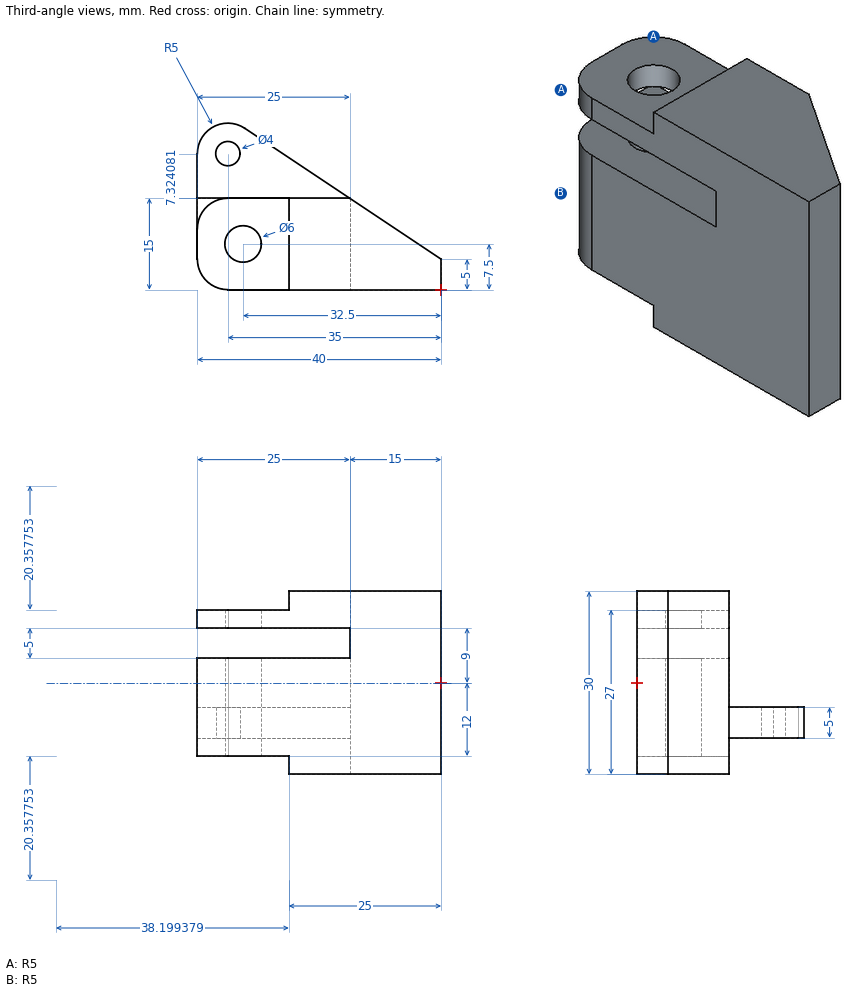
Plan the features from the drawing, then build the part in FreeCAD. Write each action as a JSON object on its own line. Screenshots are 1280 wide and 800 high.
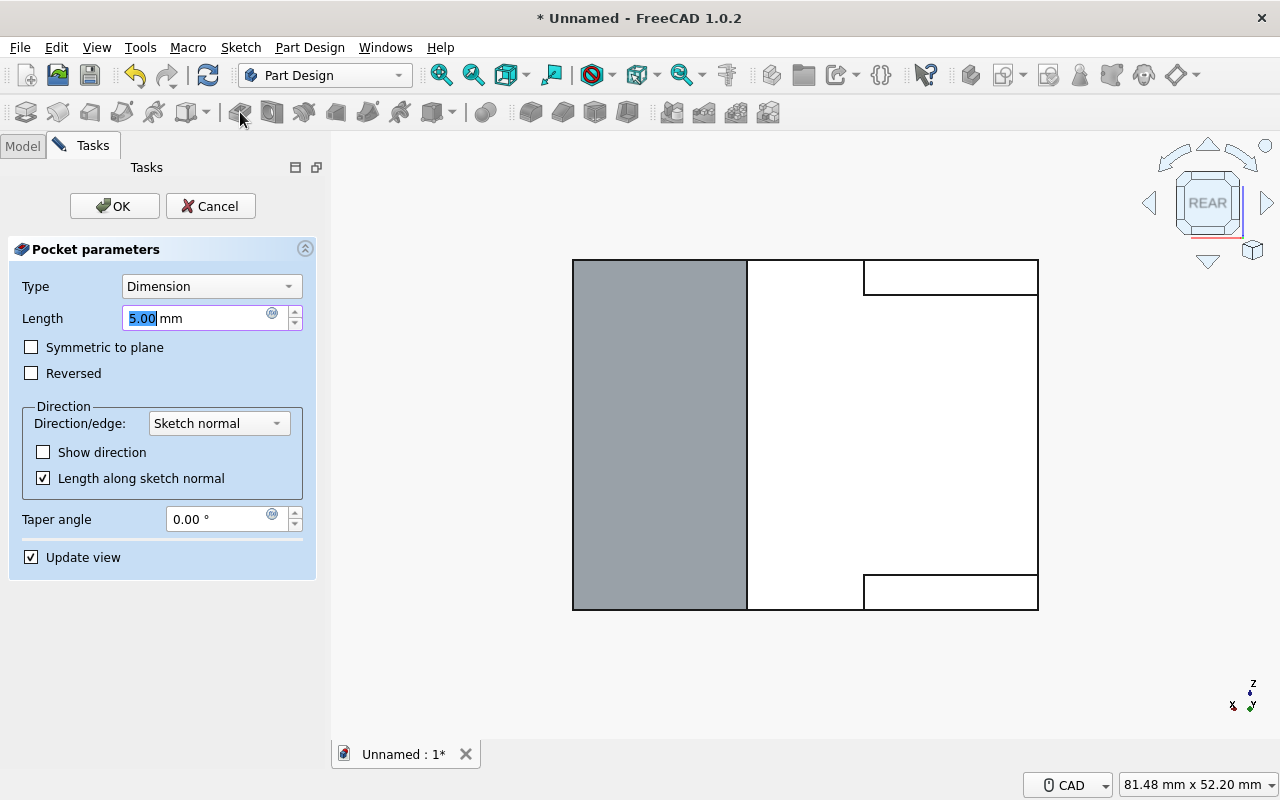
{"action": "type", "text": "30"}
{"action": "key", "text": "Tab"}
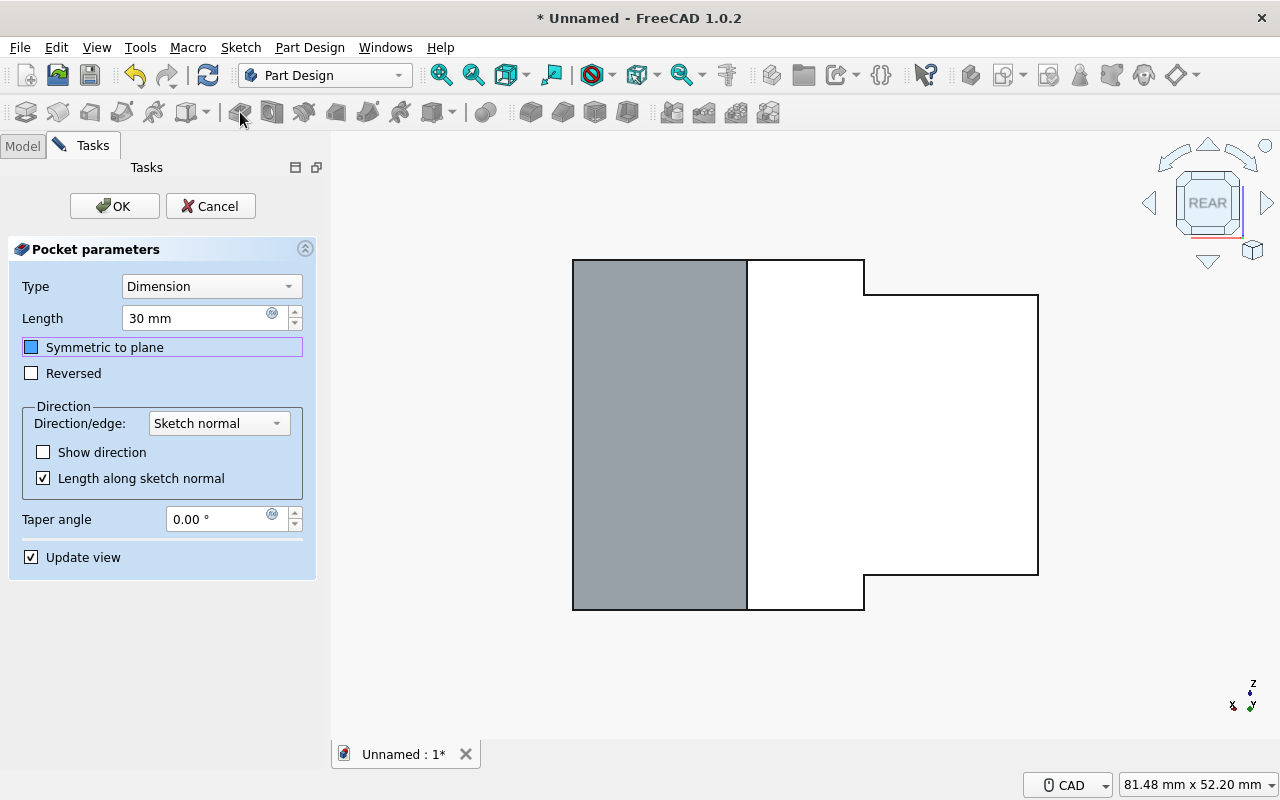
{"action": "left_click", "coordinate": [115, 206]}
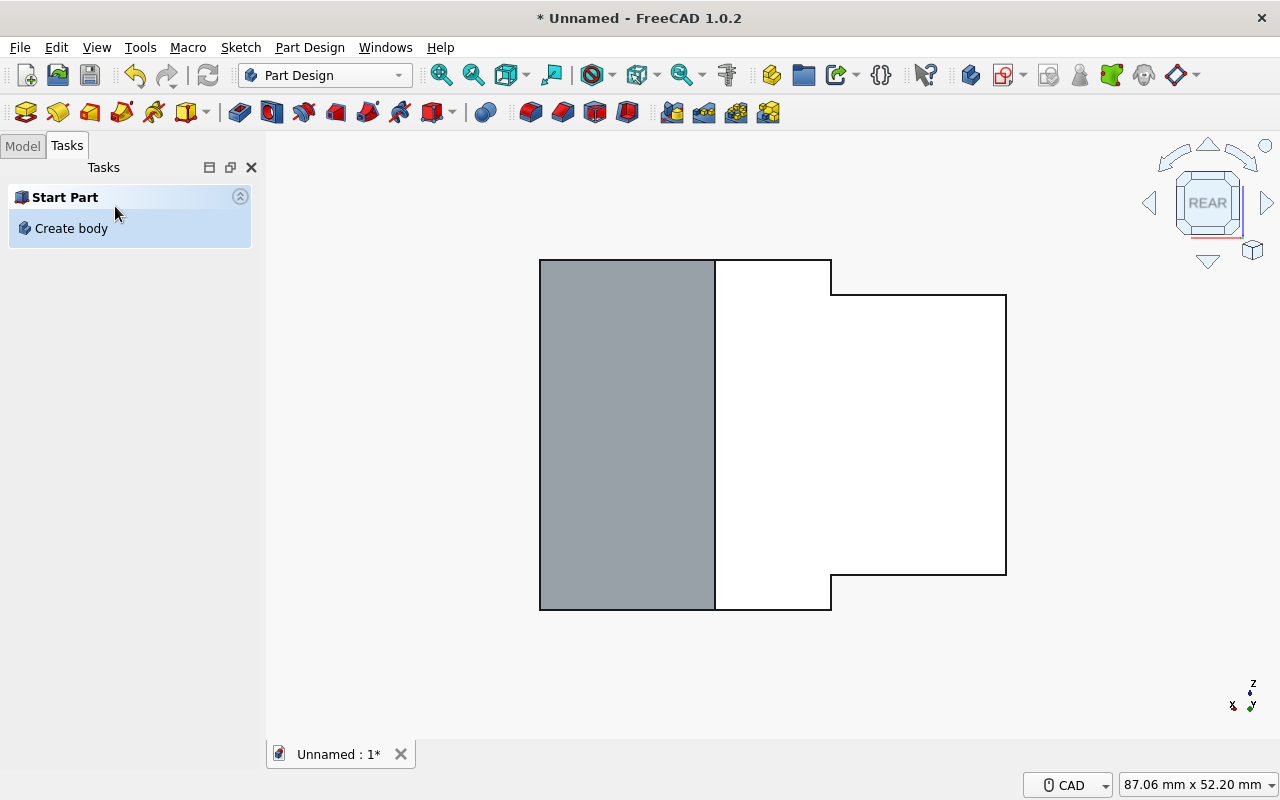
{"action": "left_click", "coordinate": [860, 434]}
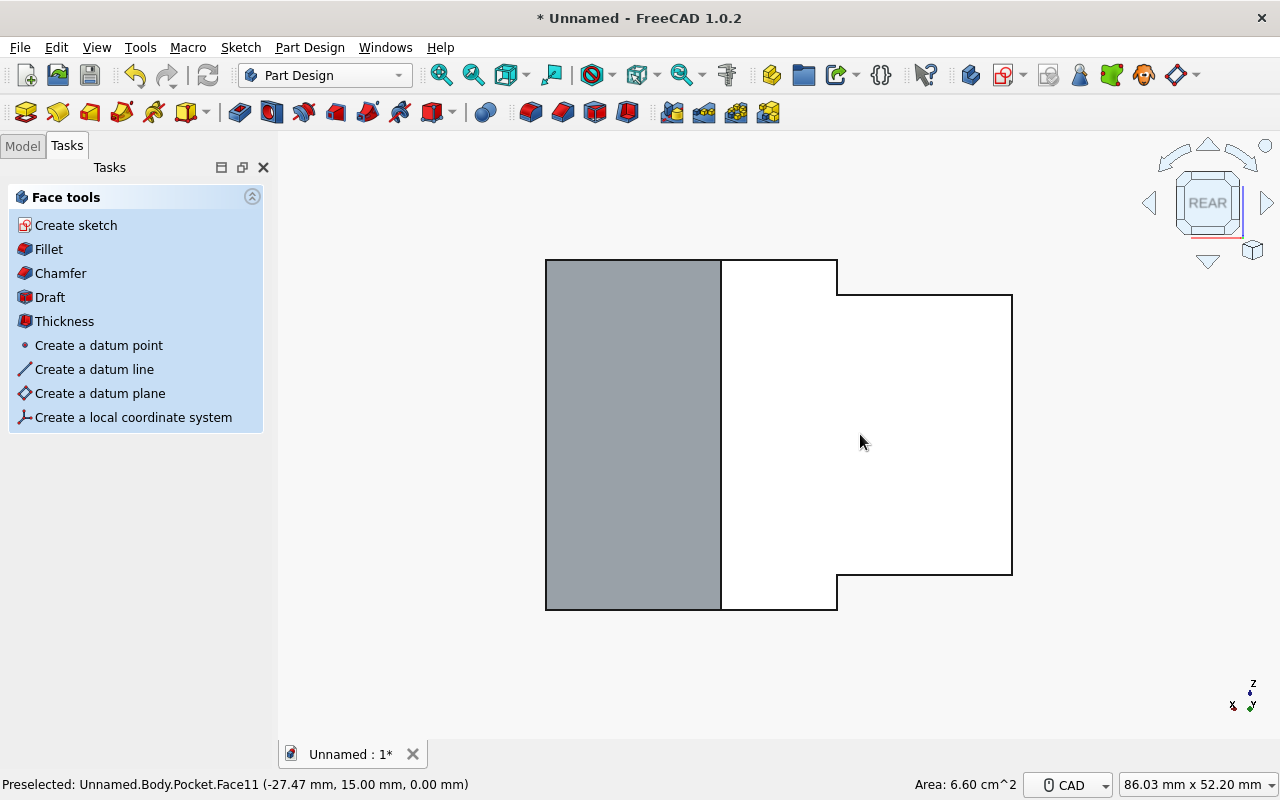
{"action": "left_click", "coordinate": [1004, 76]}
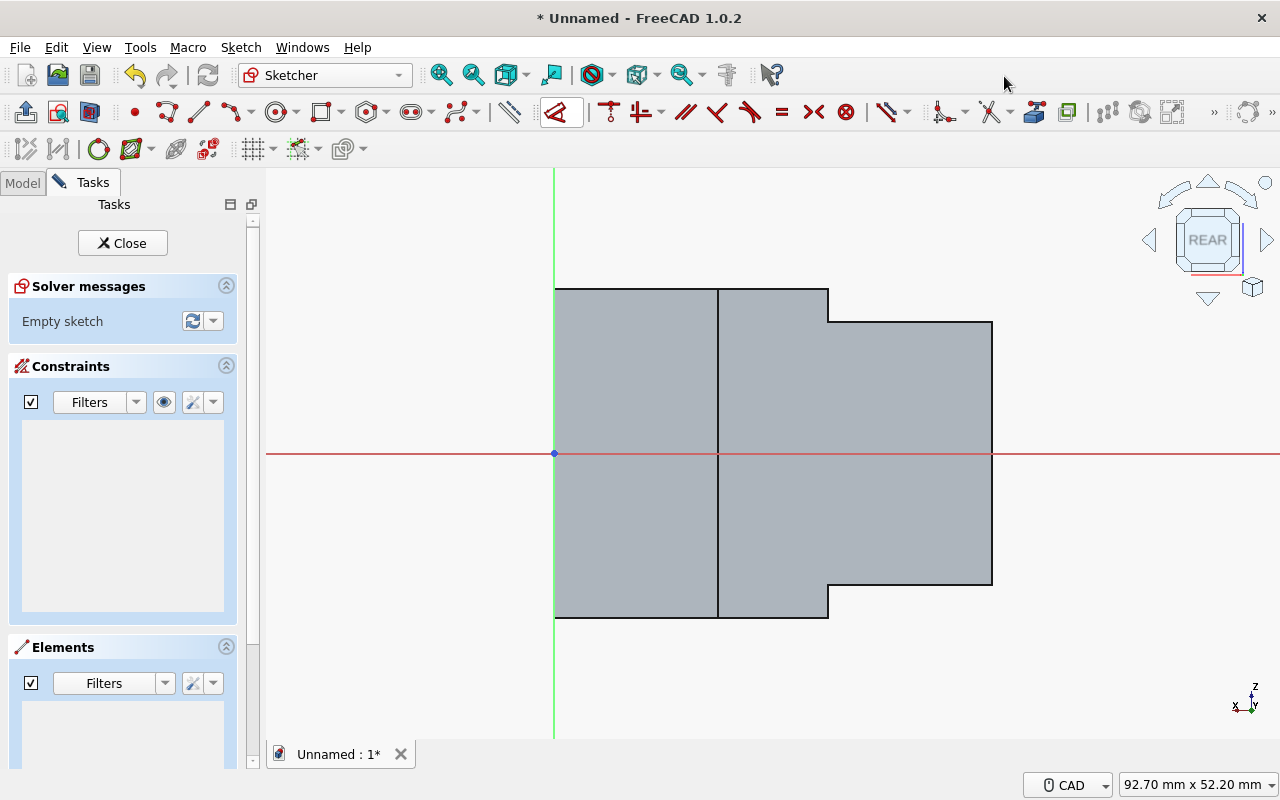
{"action": "left_click", "coordinate": [322, 112]}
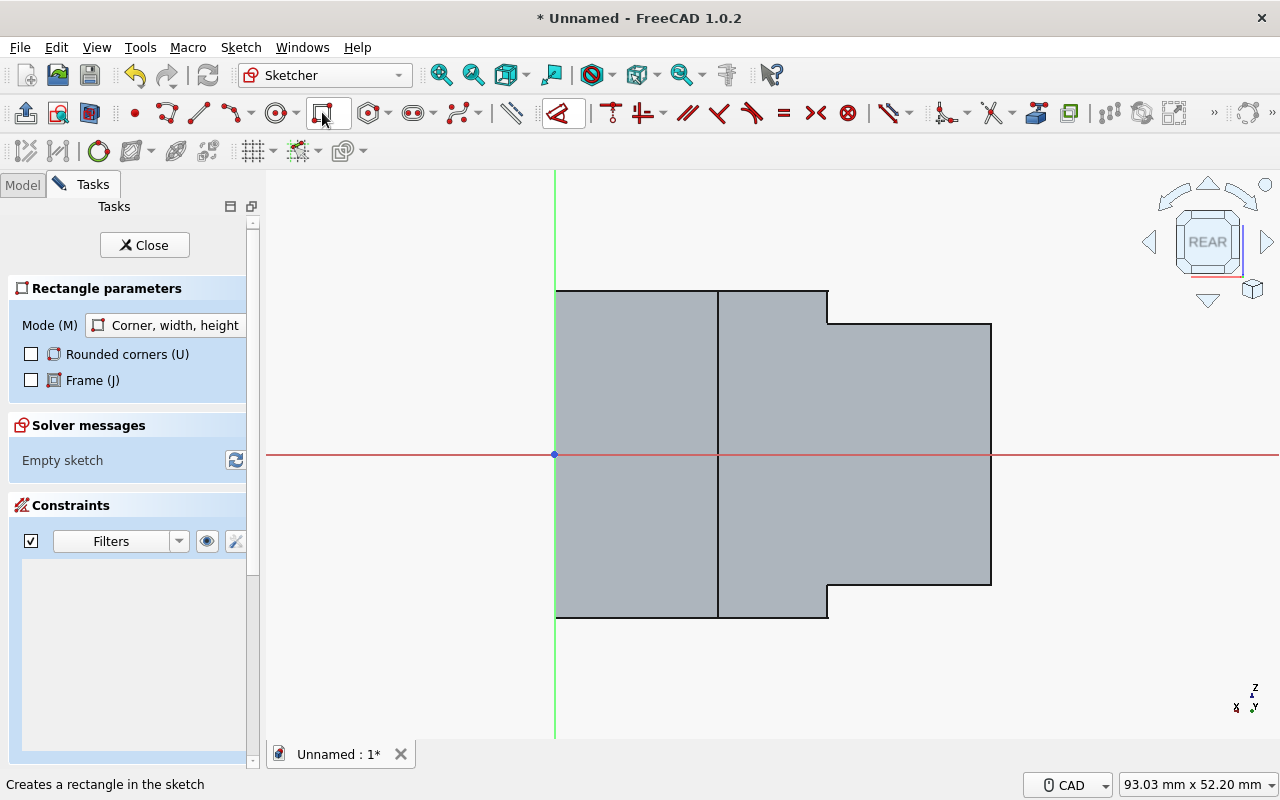
{"action": "left_click", "coordinate": [718, 356]}
{"action": "mouse_move", "coordinate": [991, 411]}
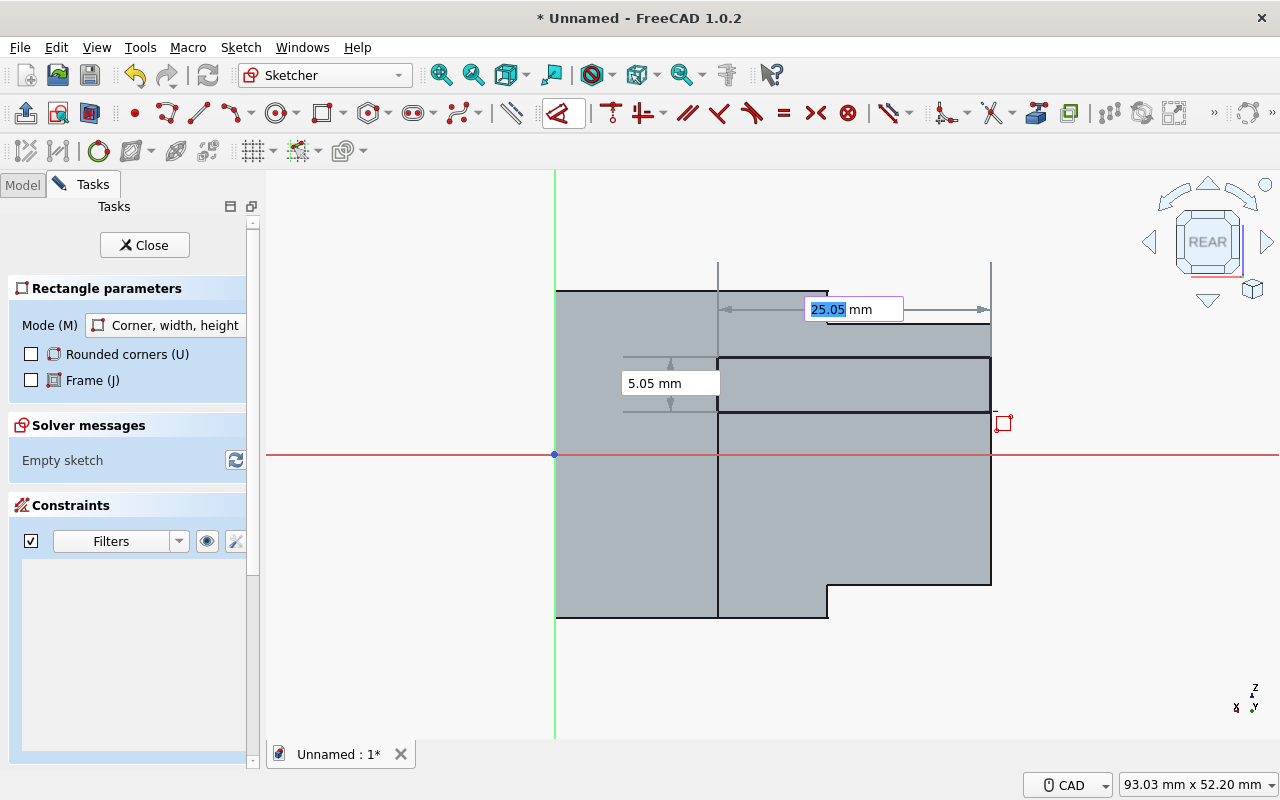
{"action": "type", "text": "25"}
{"action": "key", "text": "Tab"}
{"action": "type", "text": "5"}
{"action": "key", "text": "Return"}
{"action": "key", "text": "Escape"}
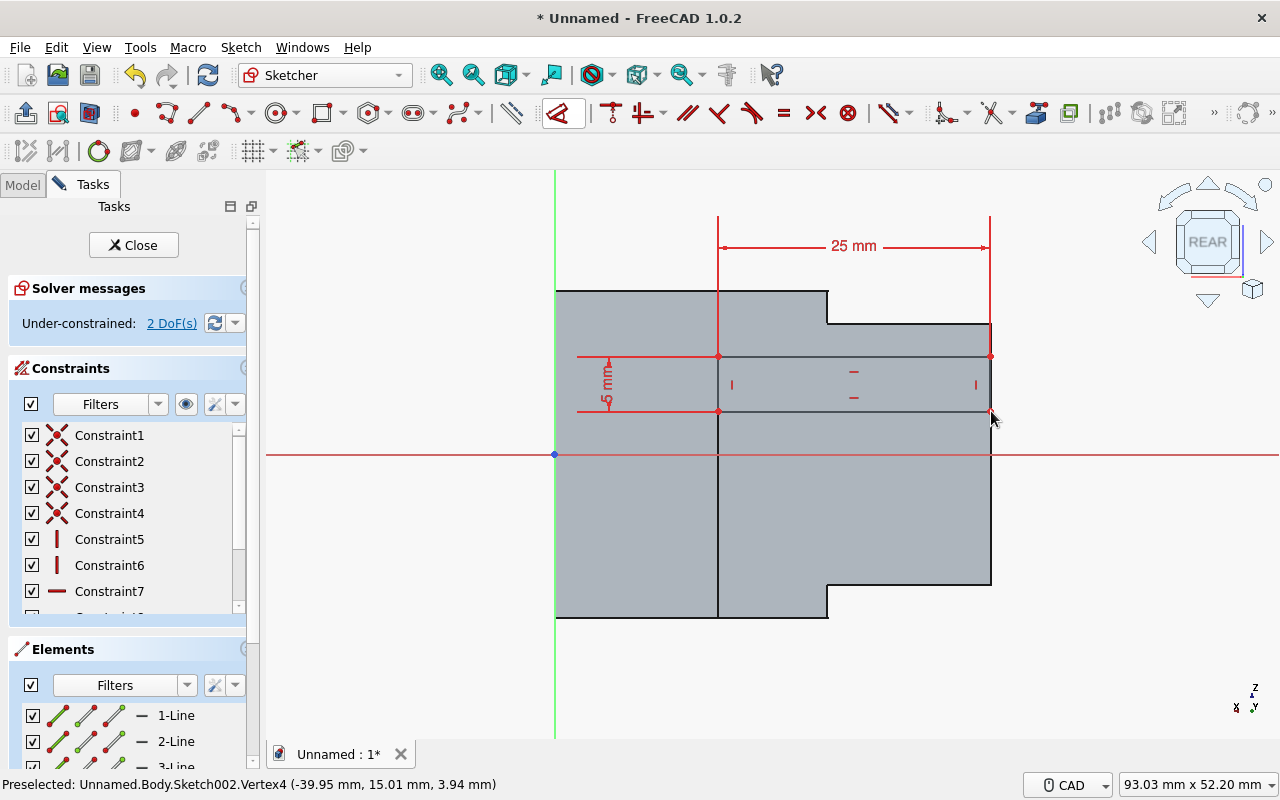
{"action": "left_click", "coordinate": [718, 357]}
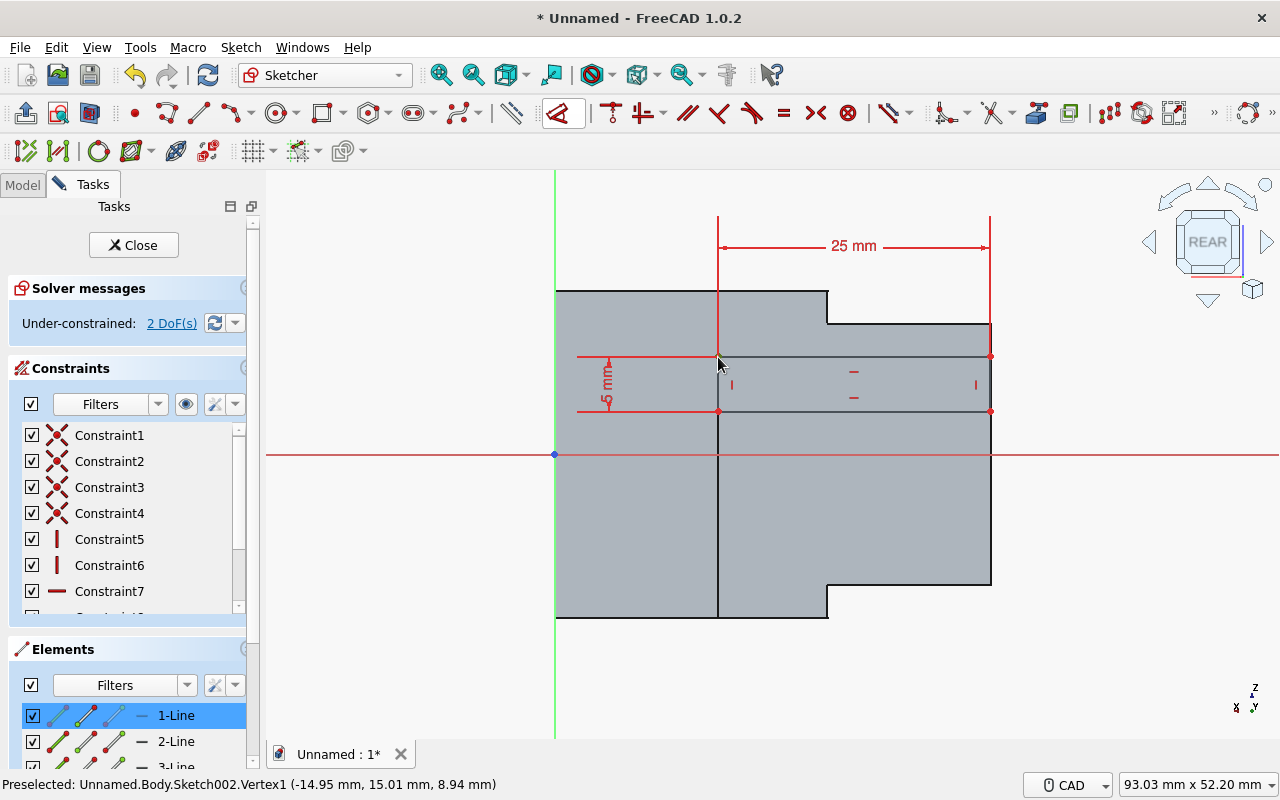
{"action": "key", "text": "i"}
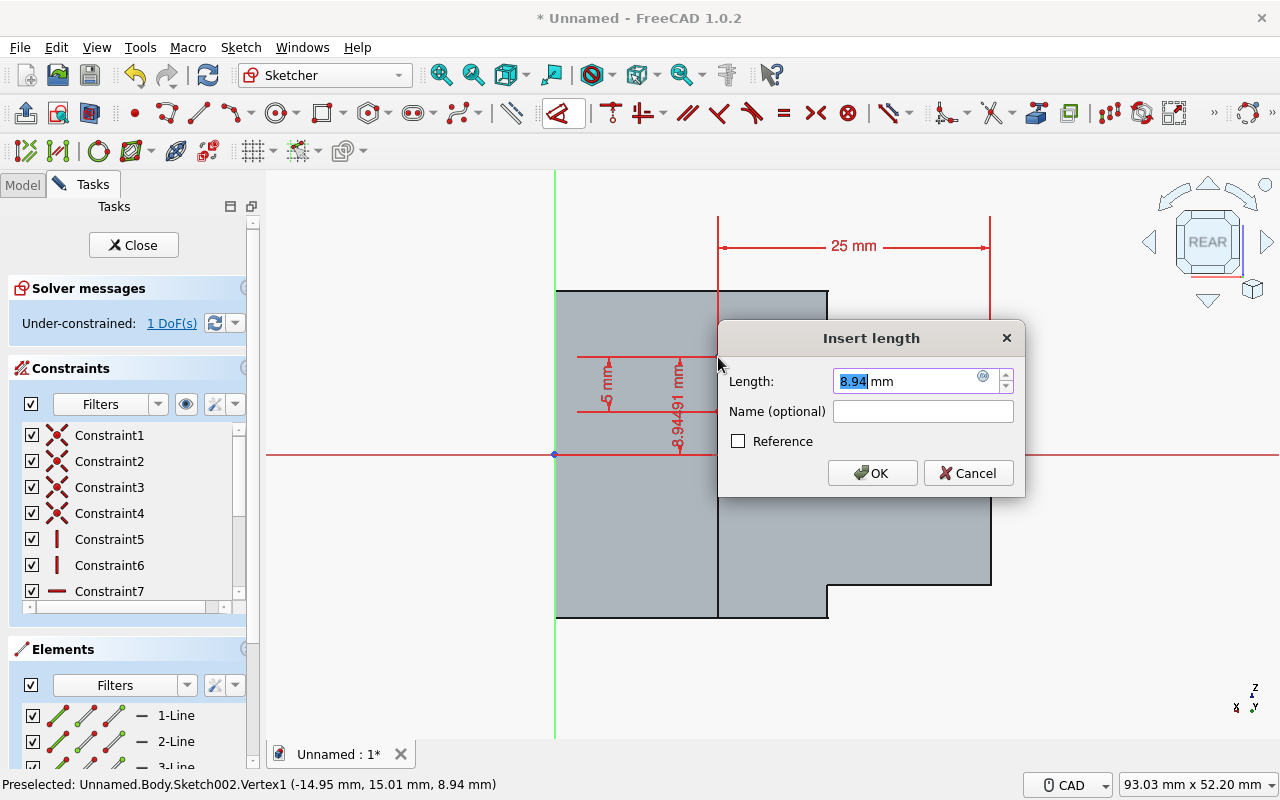
{"action": "type", "text": "9"}
{"action": "key", "text": "Return"}